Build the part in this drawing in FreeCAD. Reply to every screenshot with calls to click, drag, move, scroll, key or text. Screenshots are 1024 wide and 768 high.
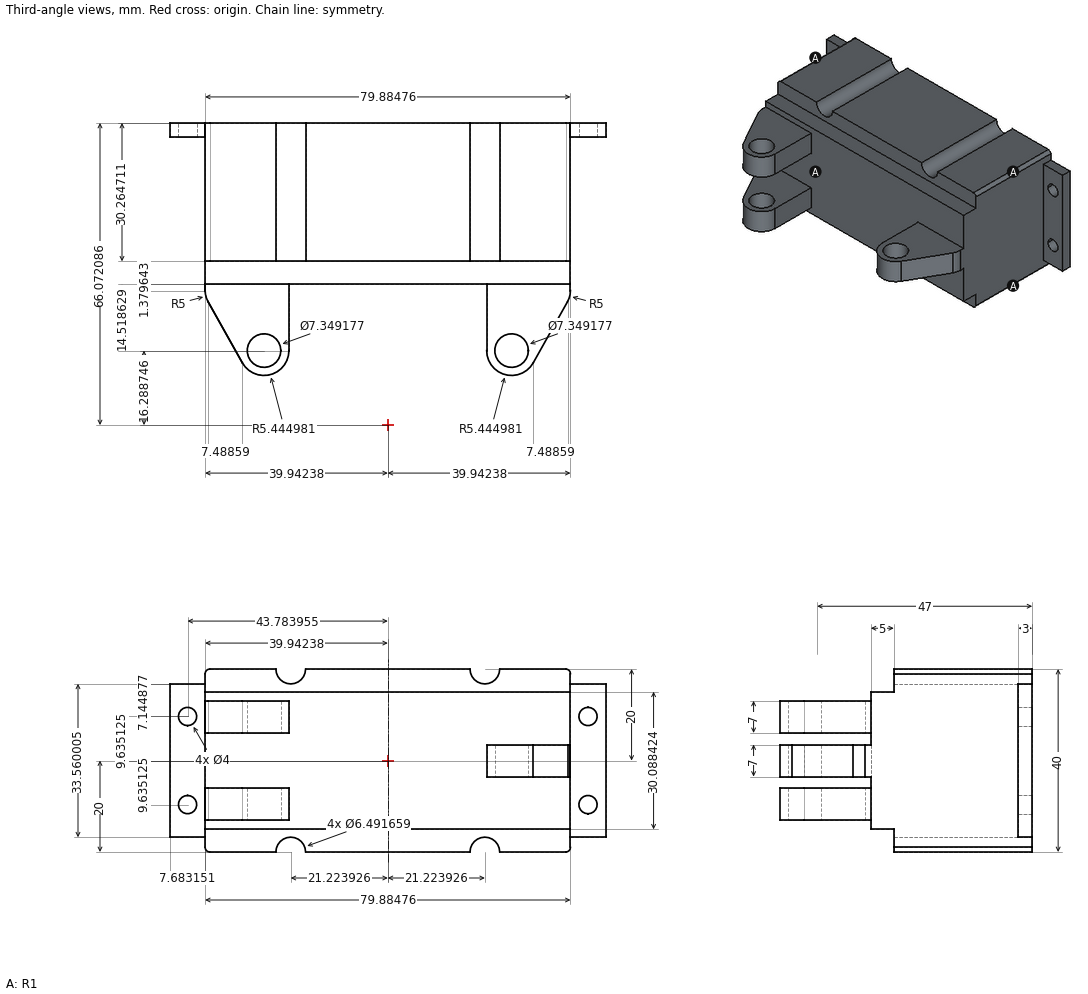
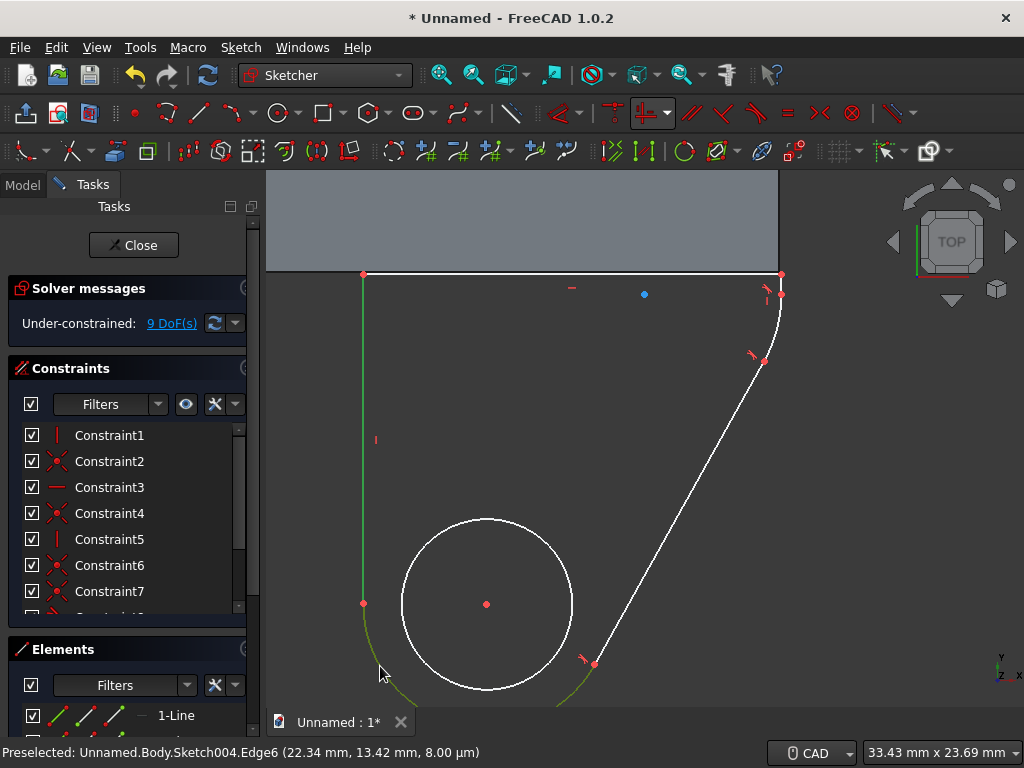
click(756, 114)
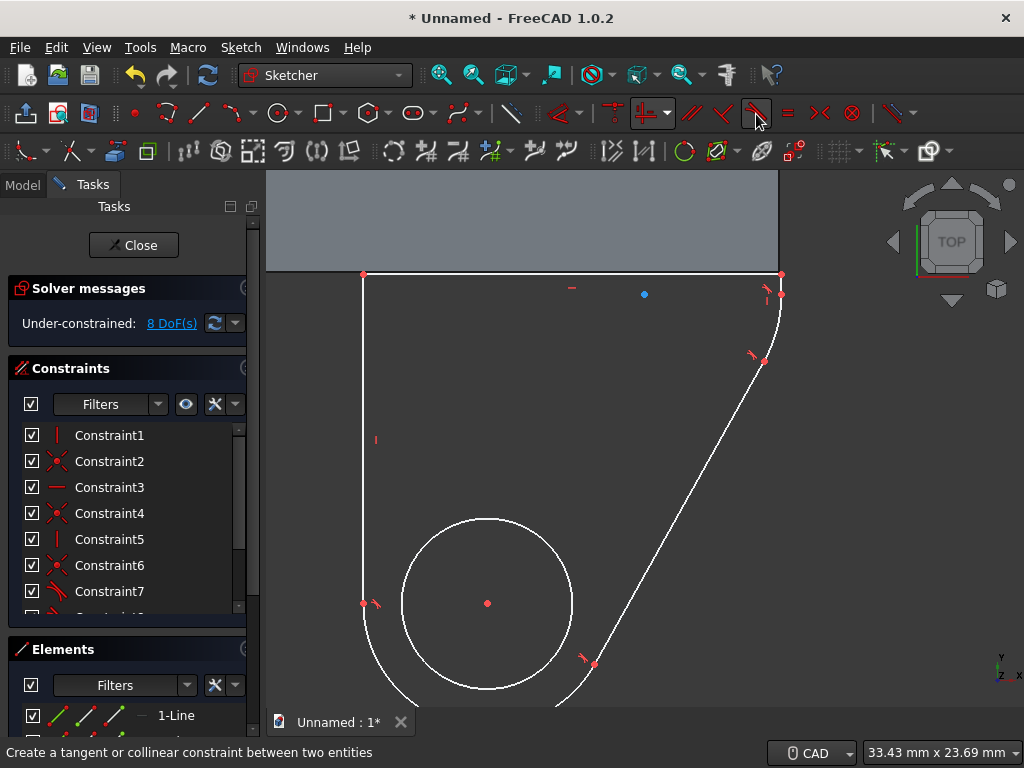
click(558, 114)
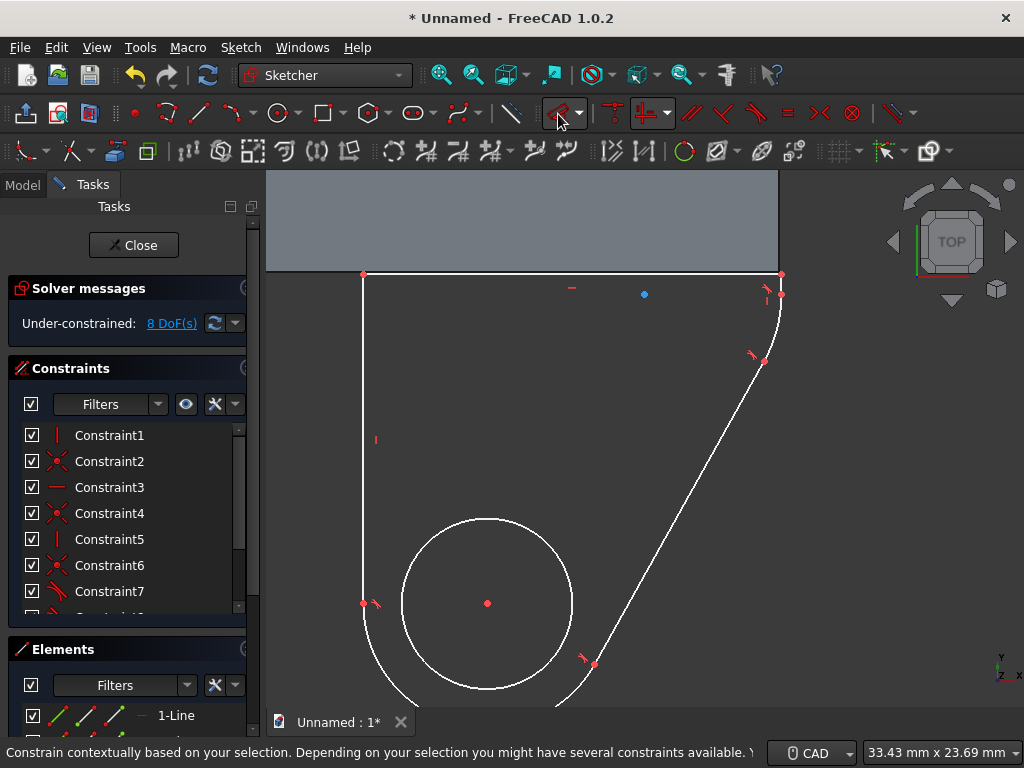
click(773, 342)
click(803, 353)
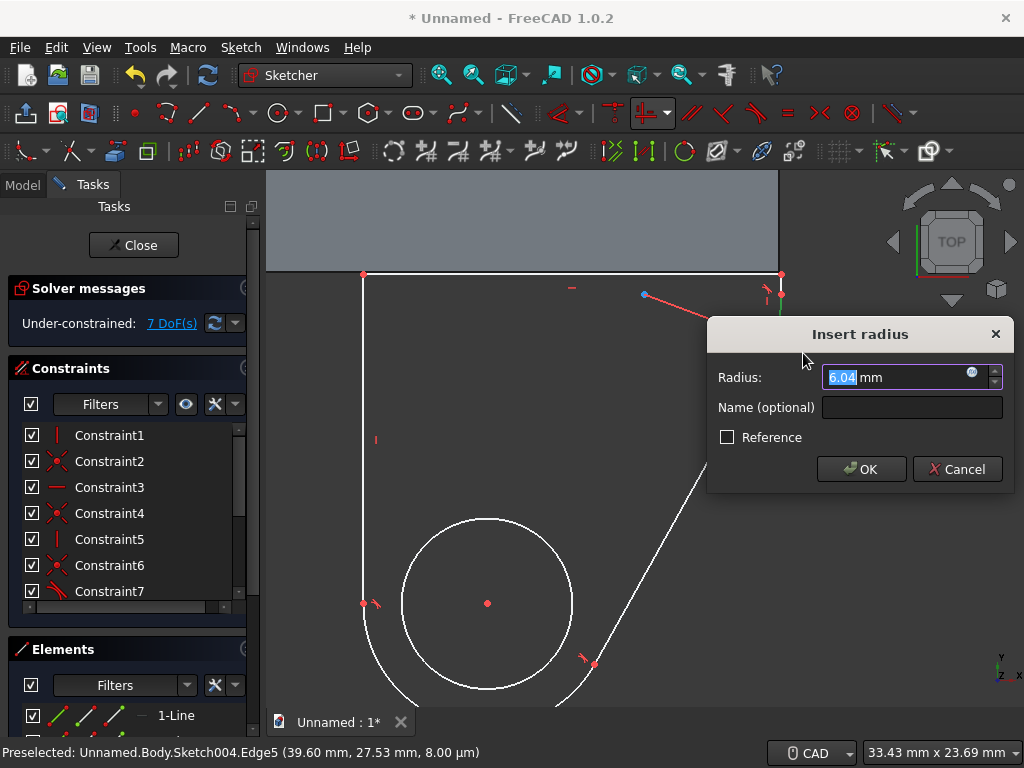
text(5)
key(Return)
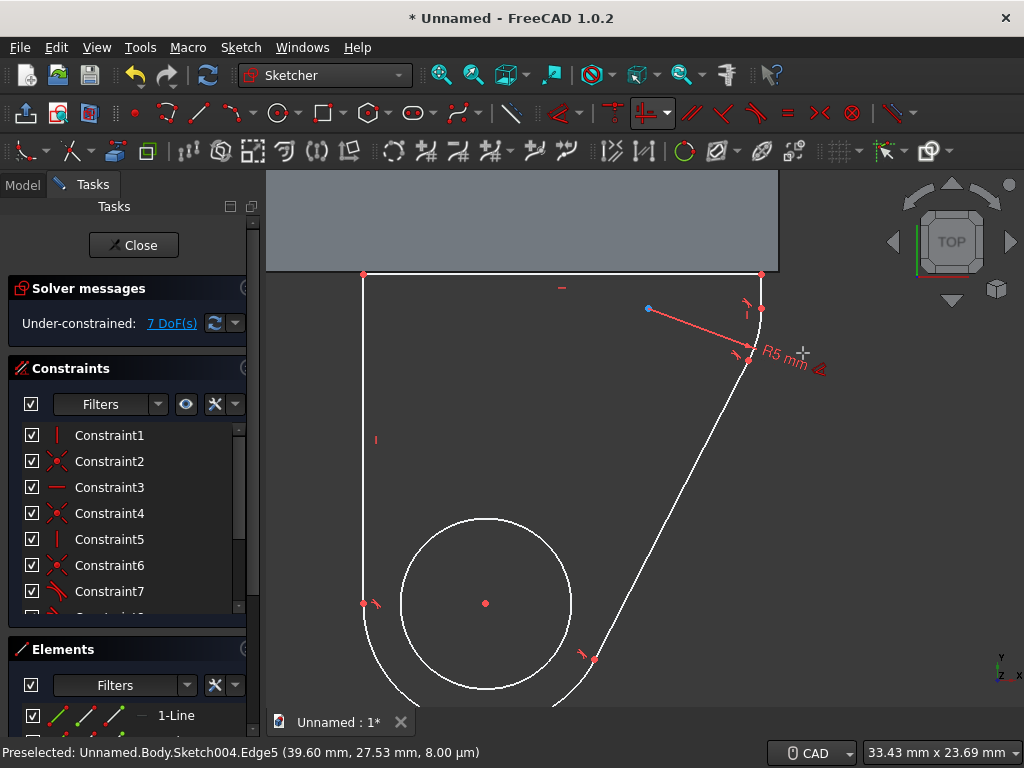
click(380, 666)
click(331, 609)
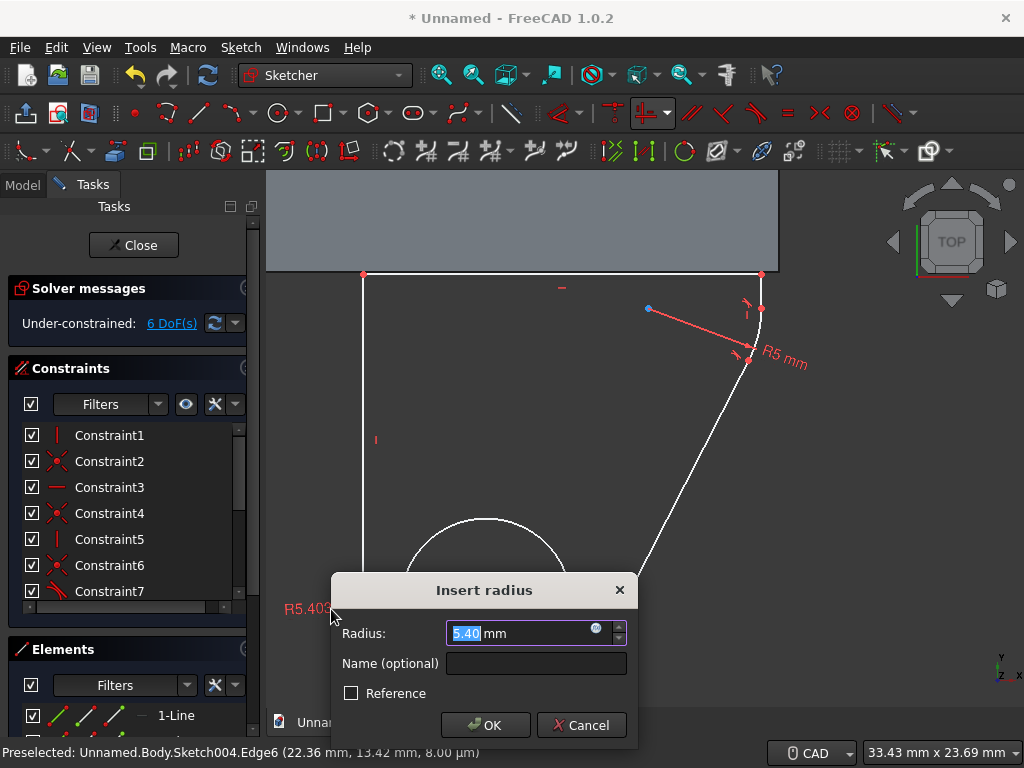
text(5.444981)
key(Return)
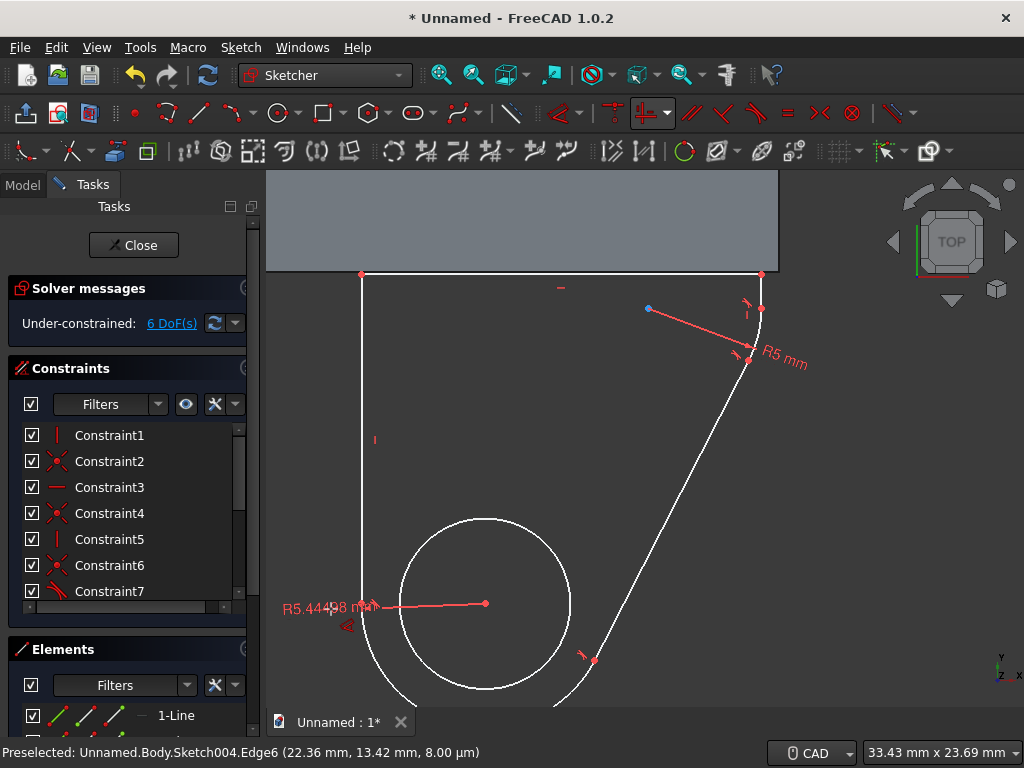
click(545, 543)
click(567, 520)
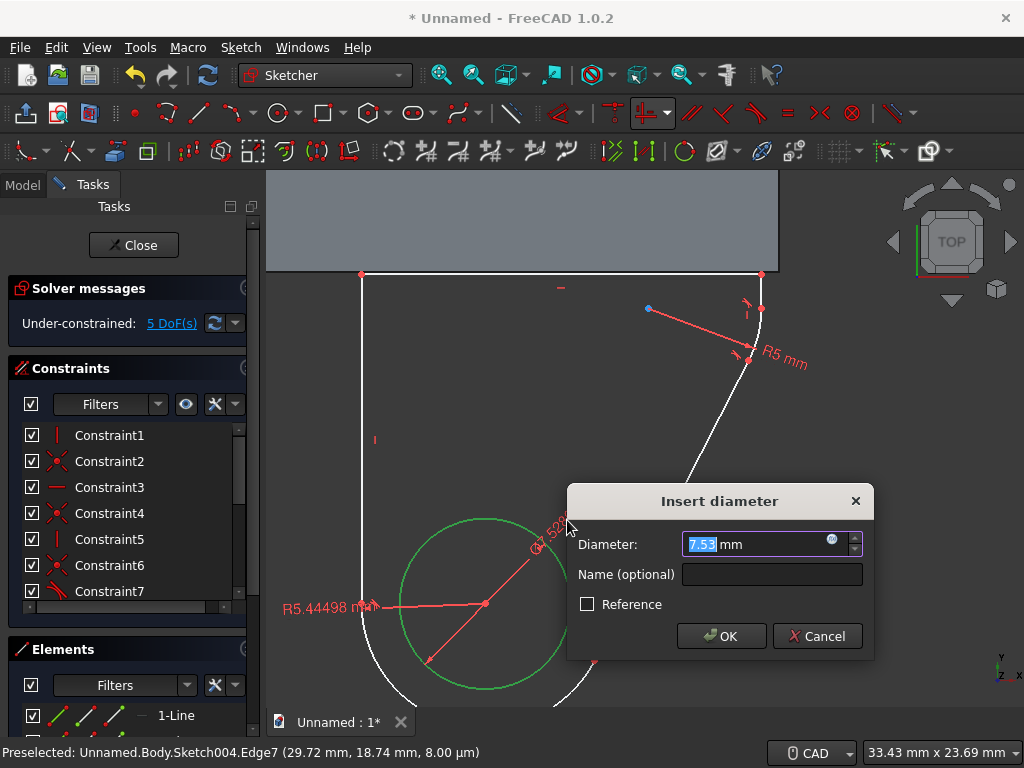
text(7.349177)
key(Return)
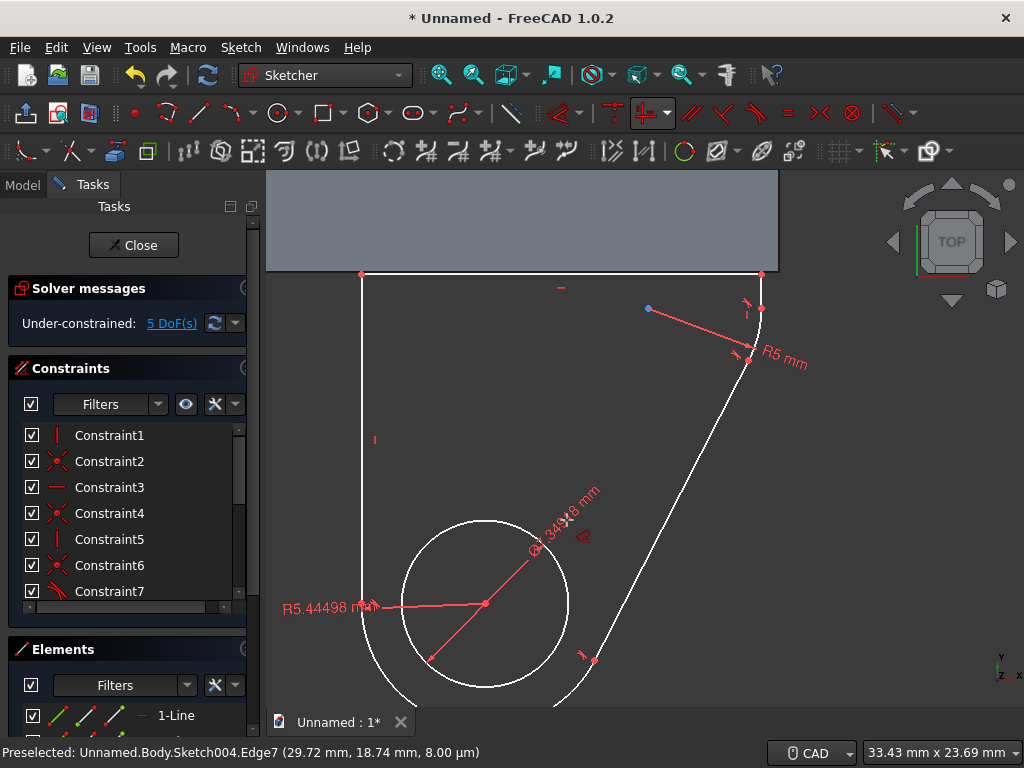
scroll(761, 298, up, 2)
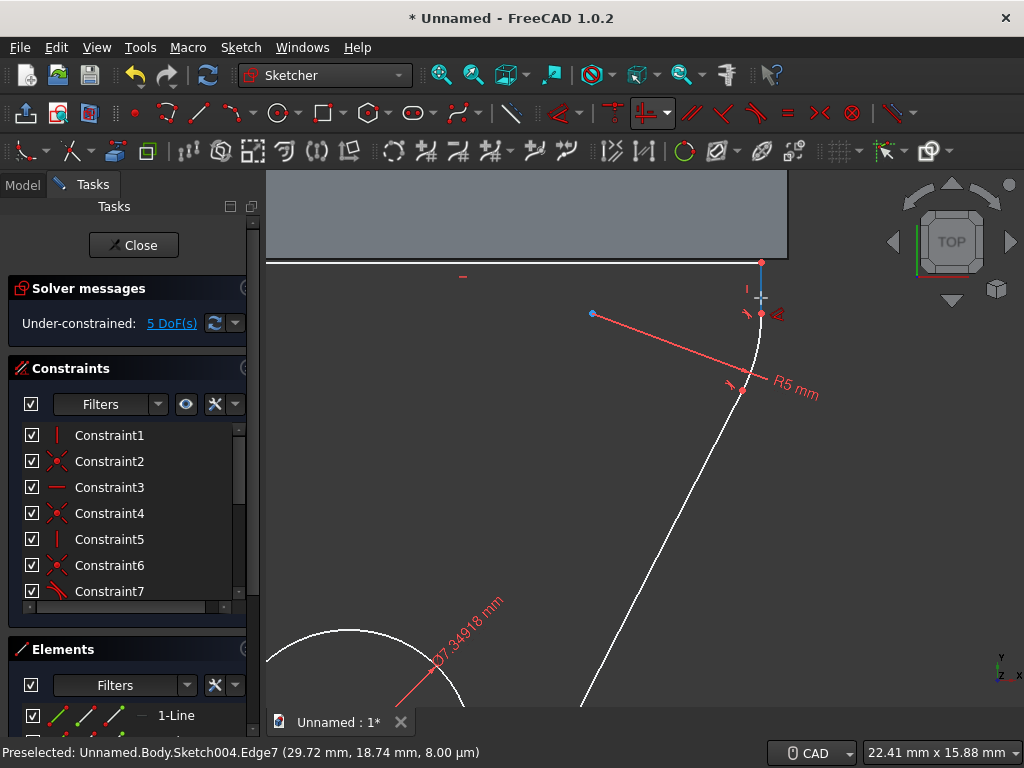
click(761, 298)
click(795, 288)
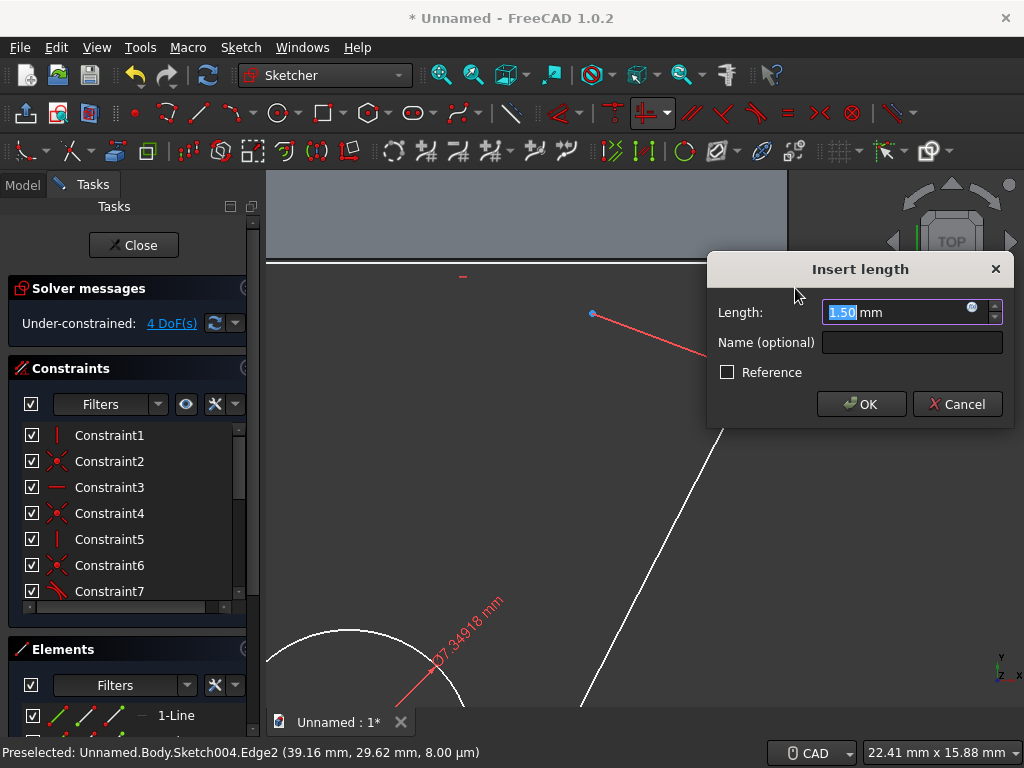
text(1.379643)
key(Return)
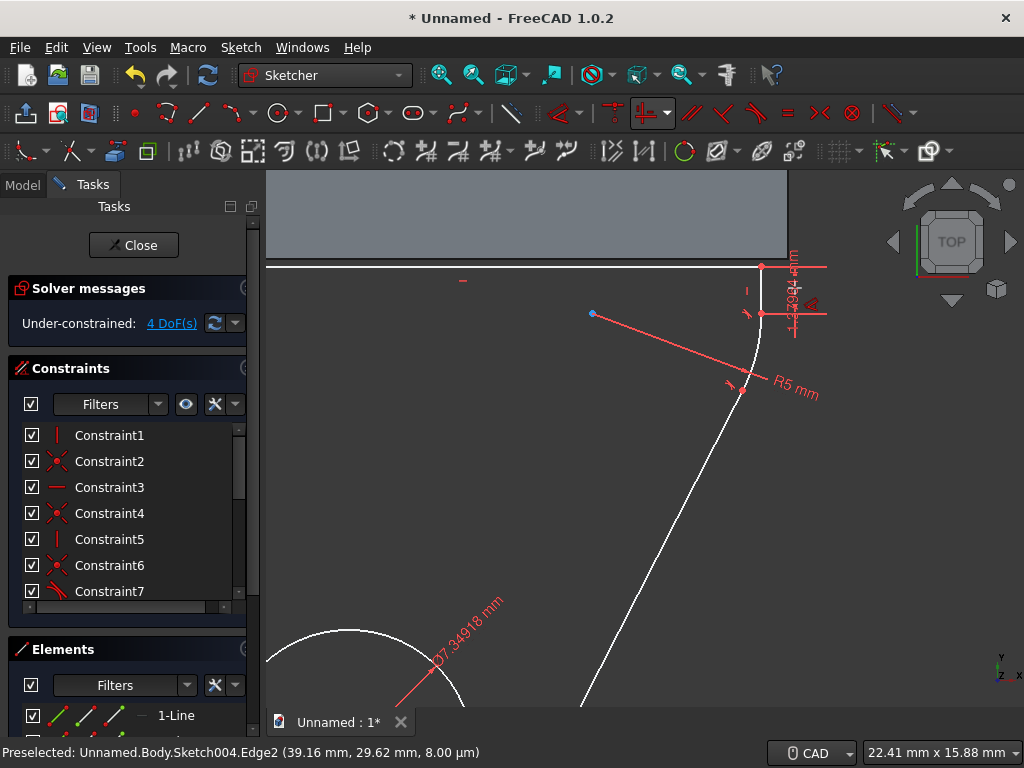
click(674, 525)
click(628, 357)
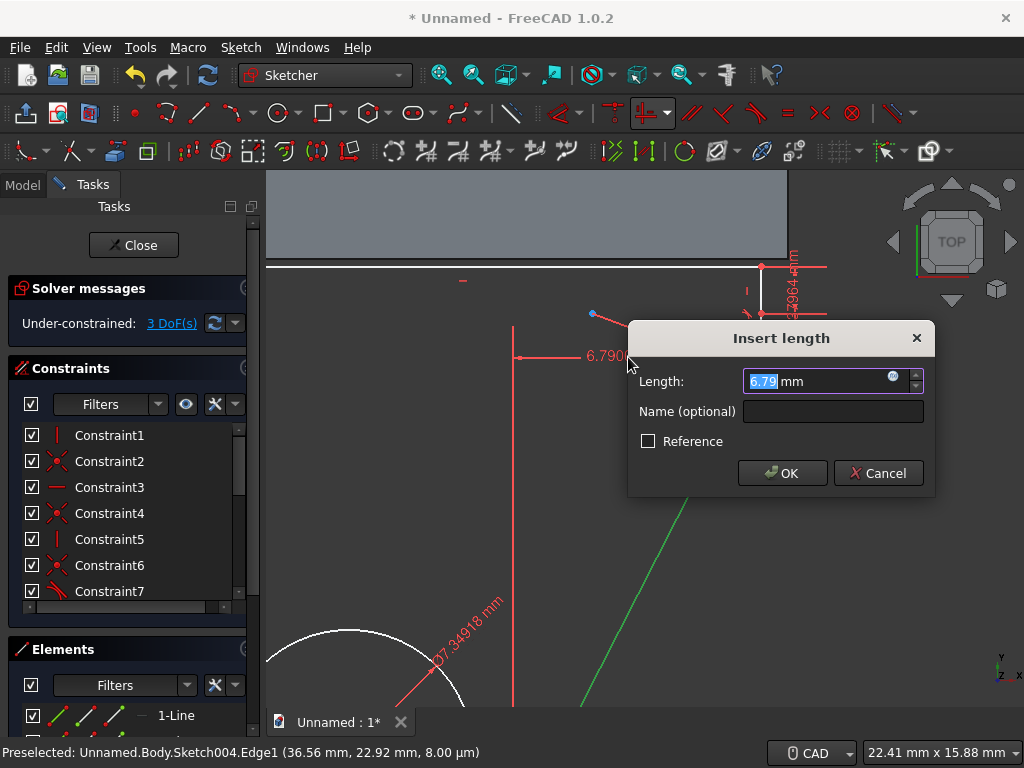
text(7.48859)
key(Return)